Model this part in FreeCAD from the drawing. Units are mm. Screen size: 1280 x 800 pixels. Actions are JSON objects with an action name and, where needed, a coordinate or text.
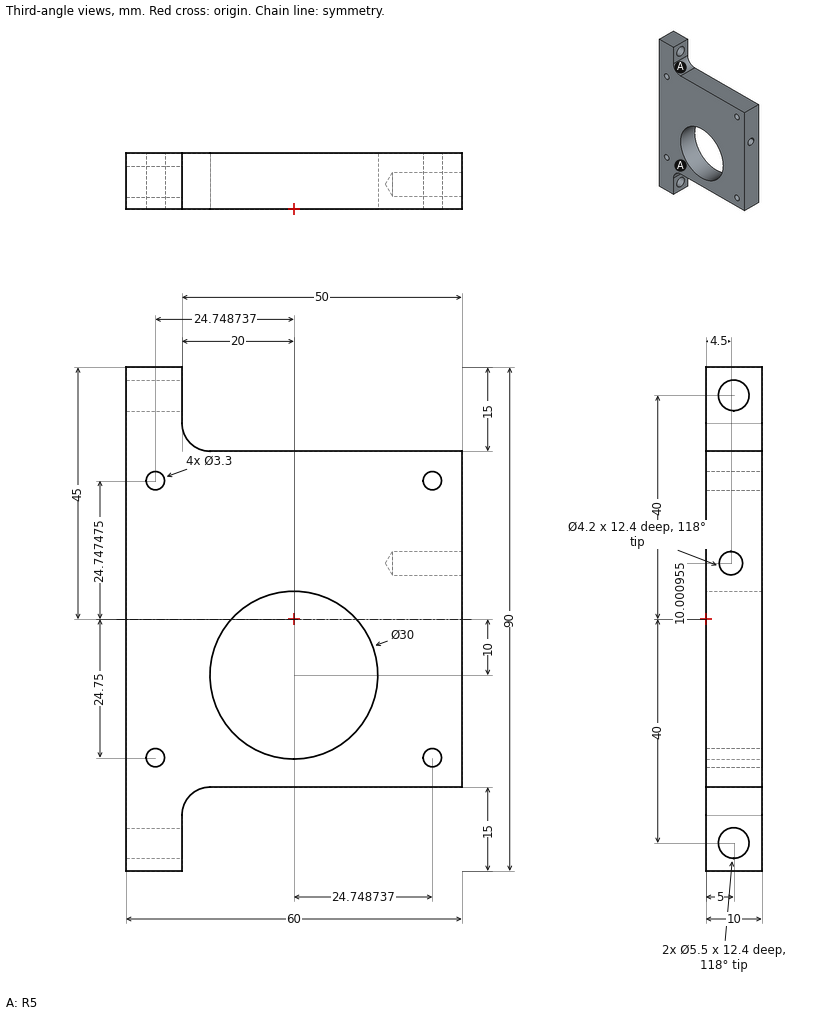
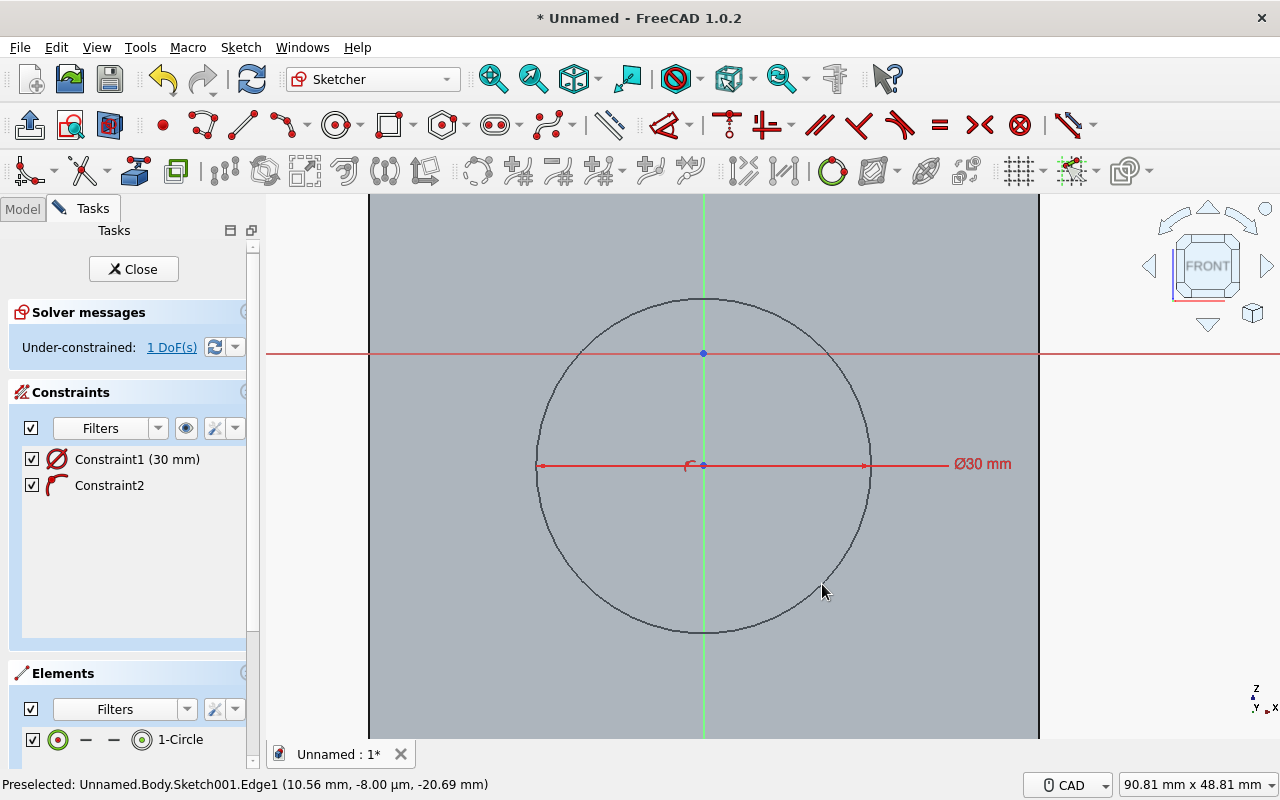
{"action": "left_click", "coordinate": [664, 126]}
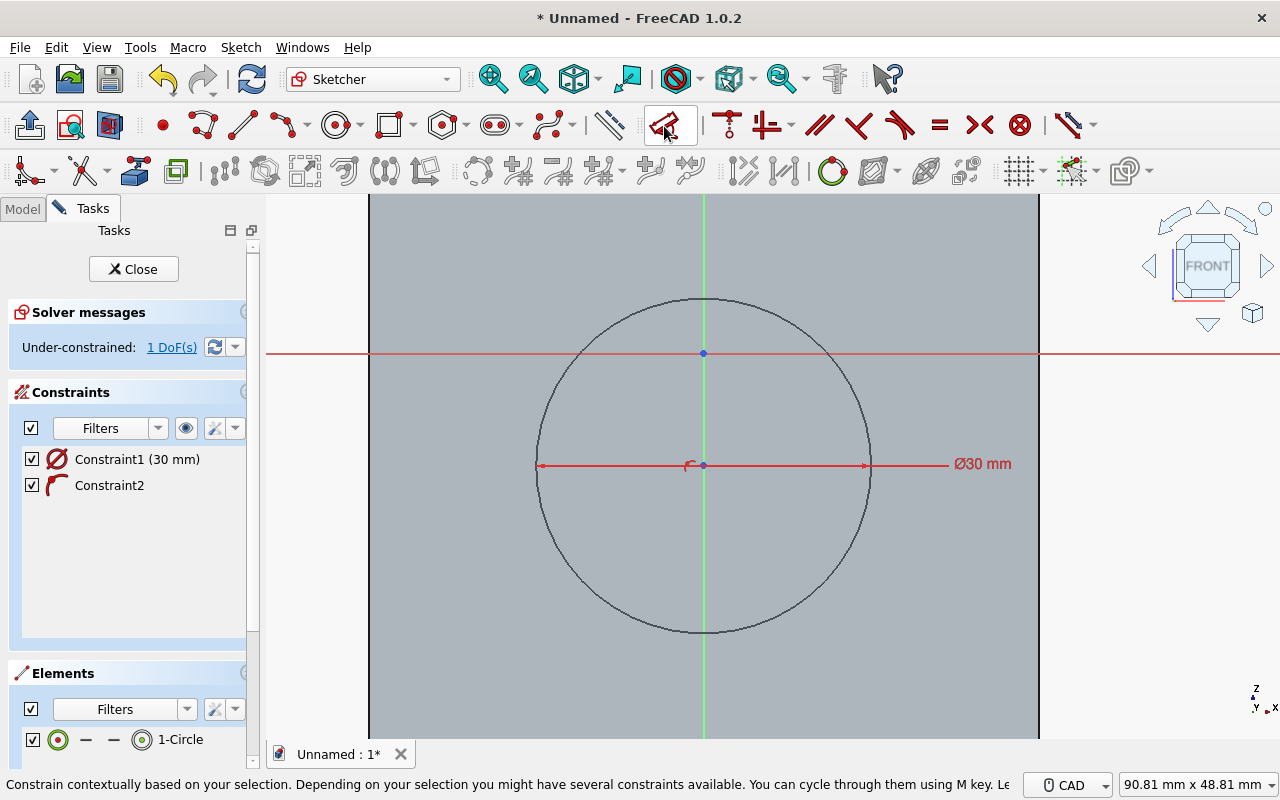
{"action": "left_click", "coordinate": [704, 466]}
{"action": "left_click", "coordinate": [738, 410]}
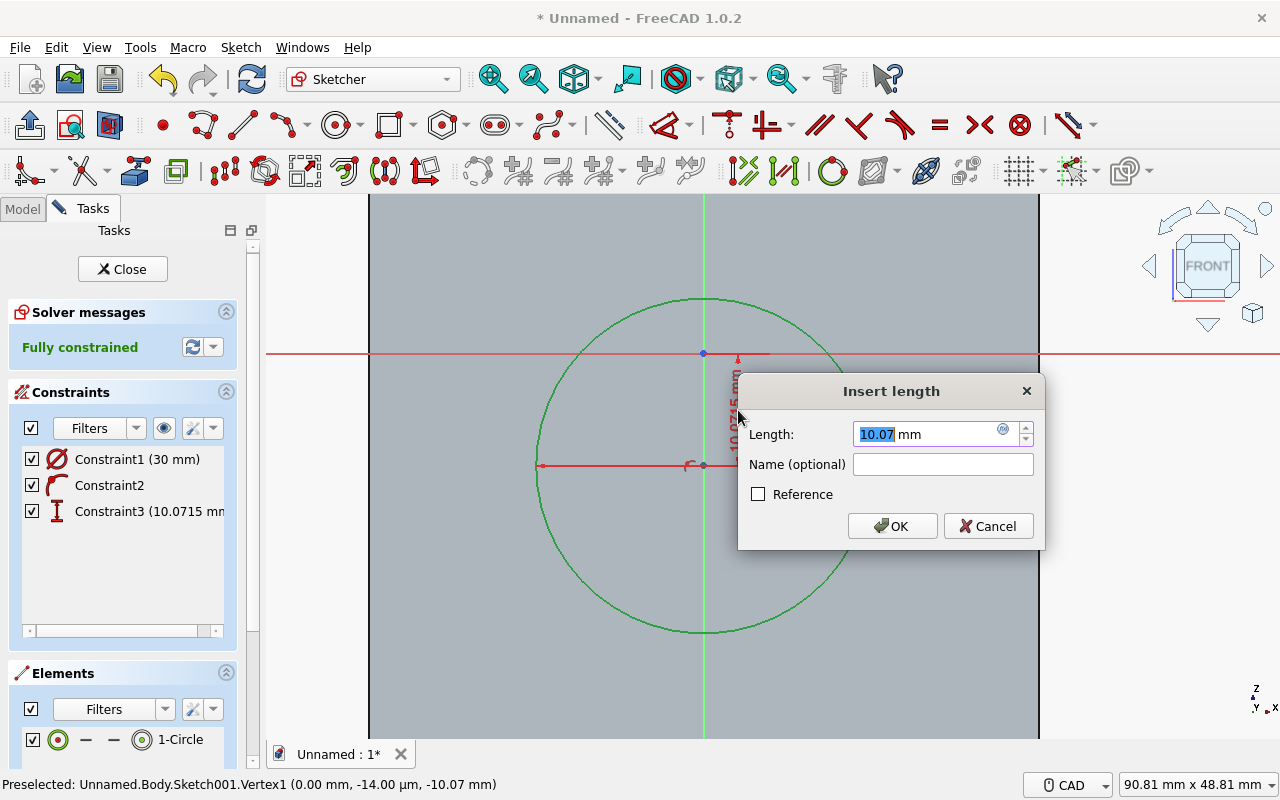
{"action": "type", "text": "10"}
{"action": "key", "text": "Return"}
{"action": "key", "text": "Escape"}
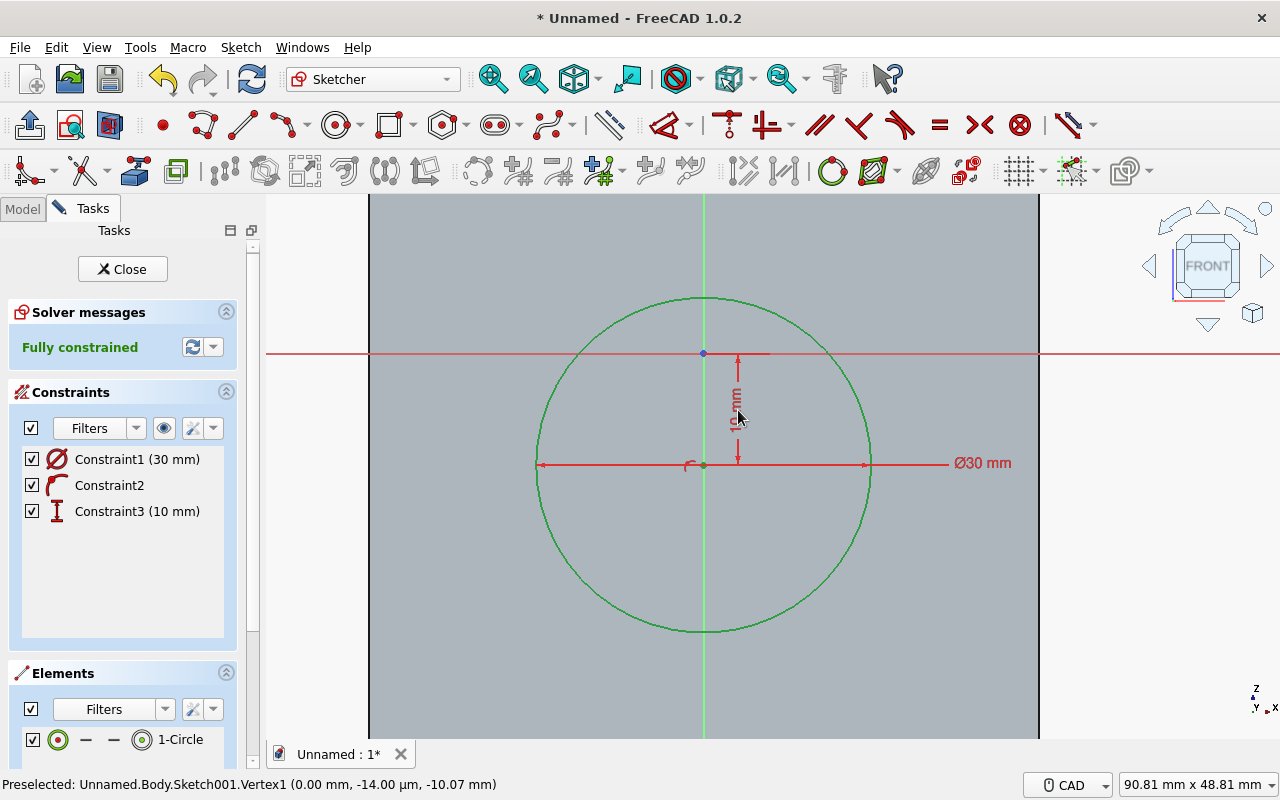
{"action": "left_click", "coordinate": [123, 269]}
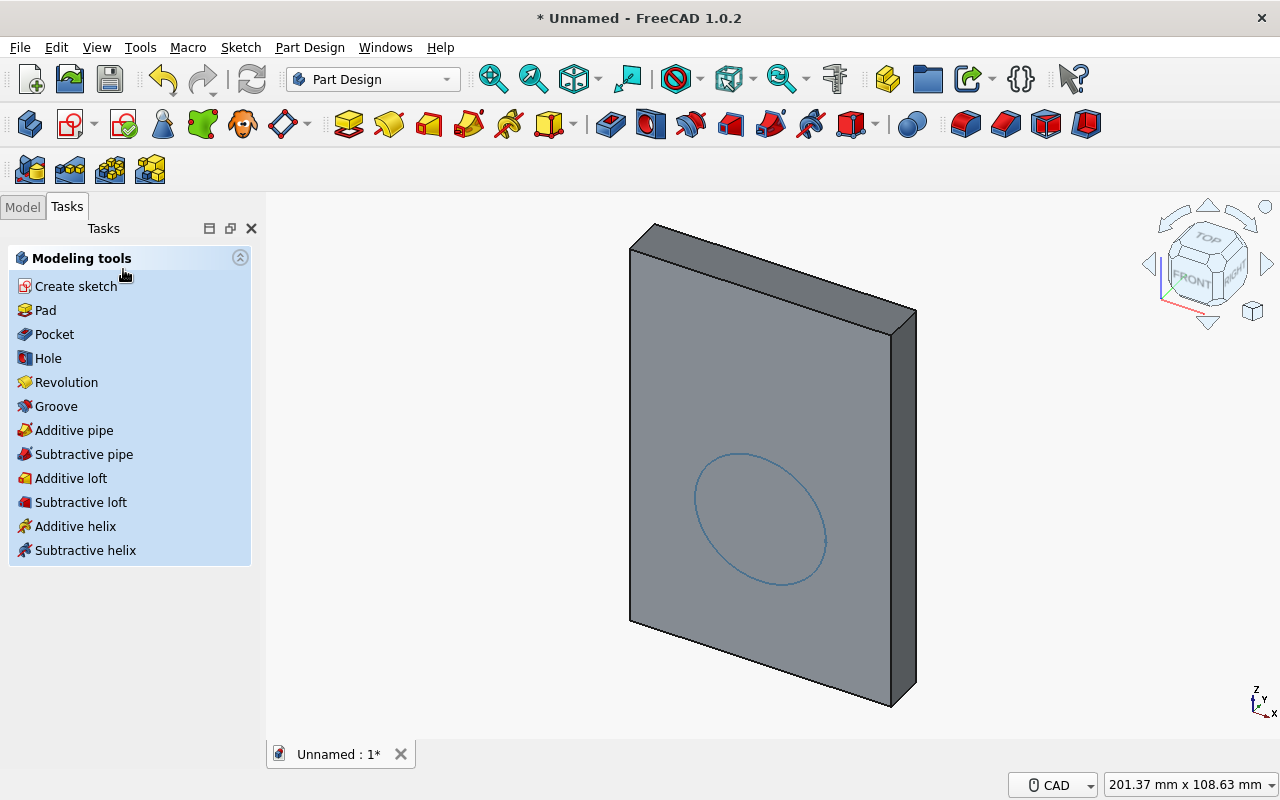
{"action": "left_click", "coordinate": [612, 124]}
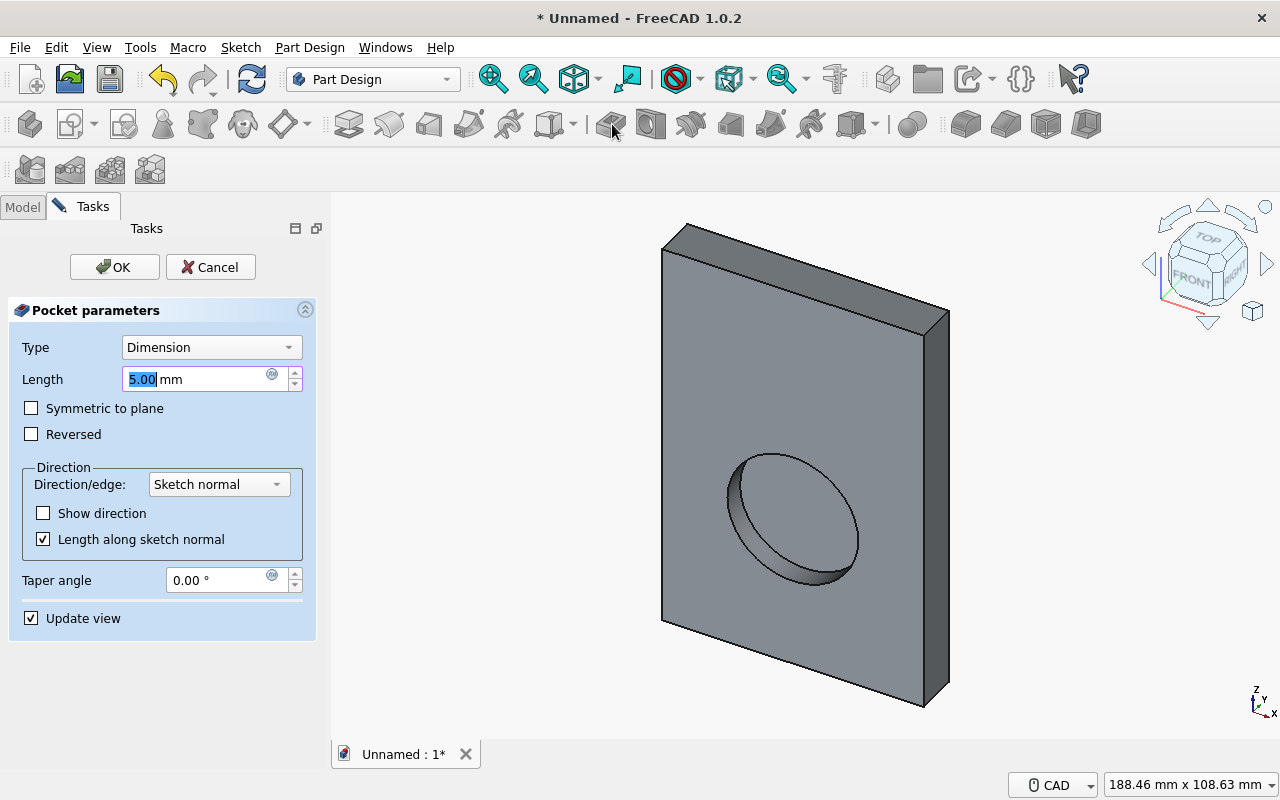
{"action": "left_click", "coordinate": [212, 348]}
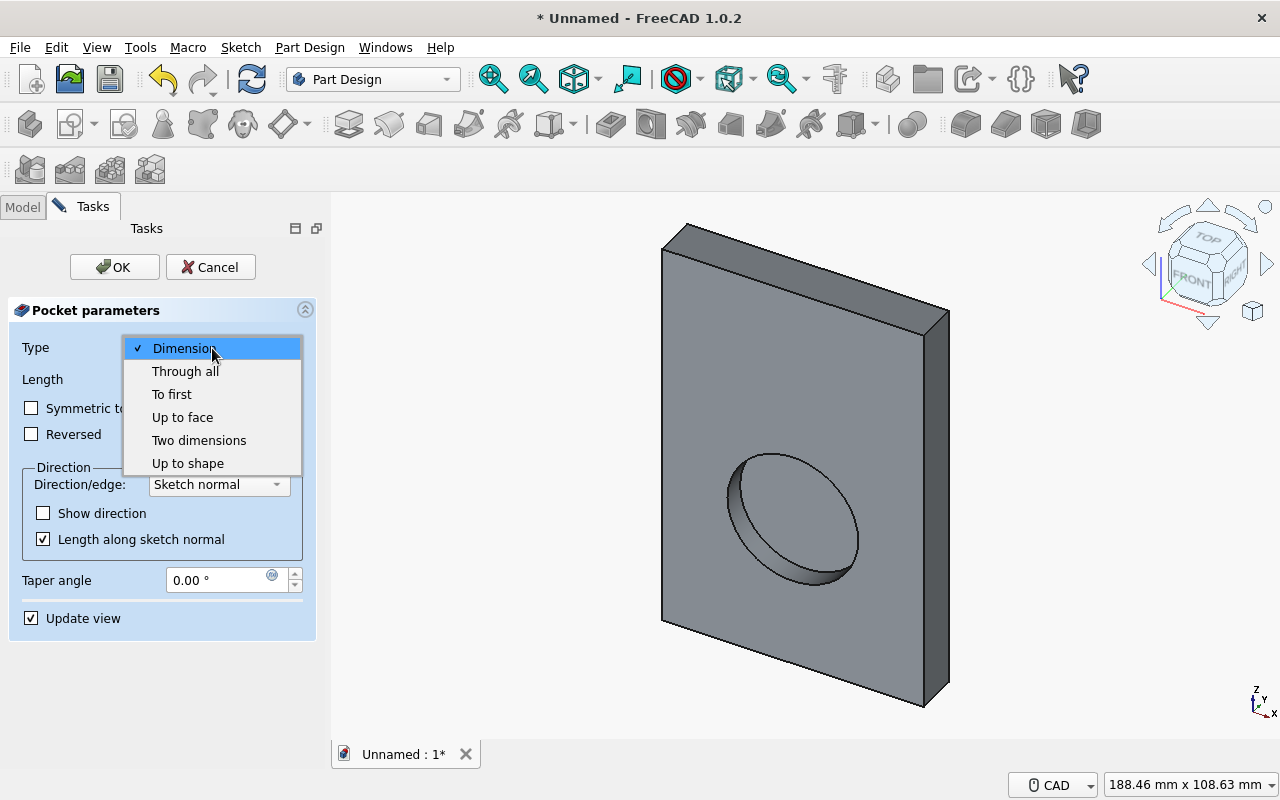
{"action": "left_click", "coordinate": [212, 372]}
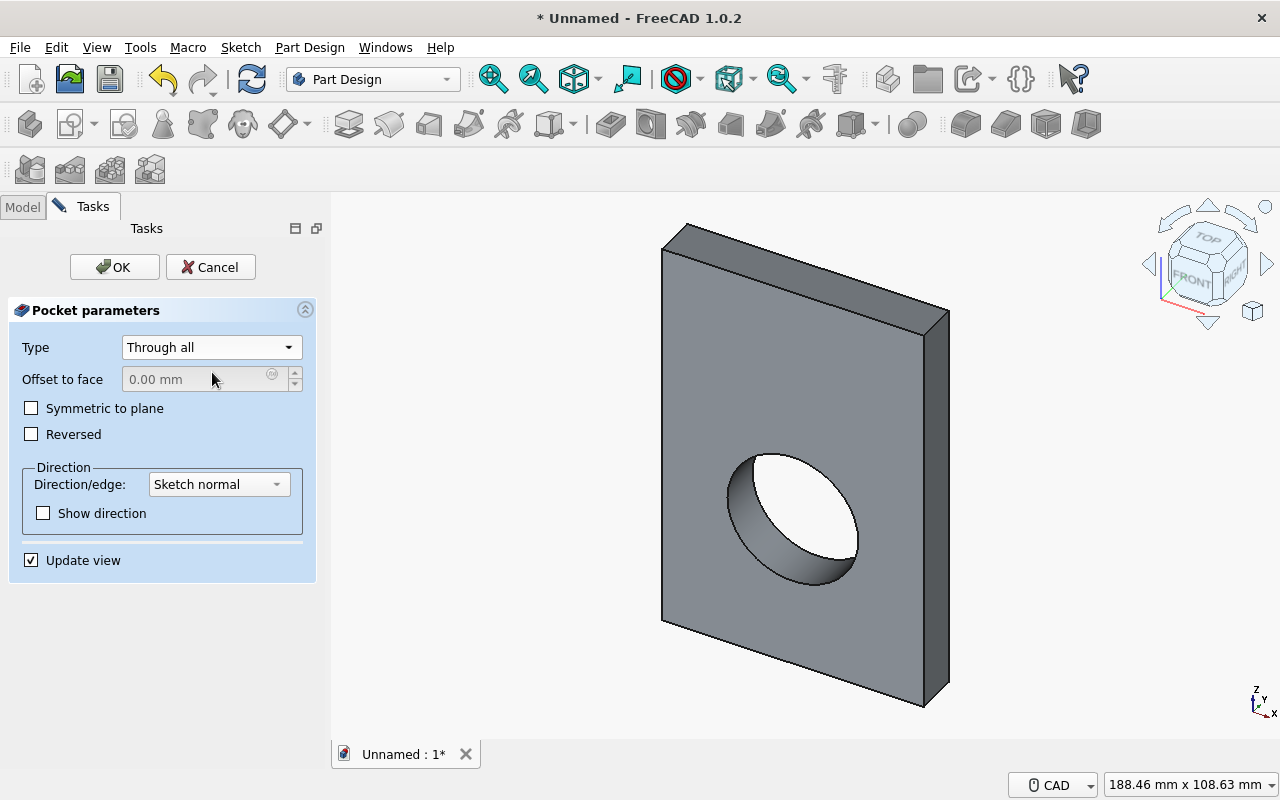
{"action": "left_click", "coordinate": [115, 267]}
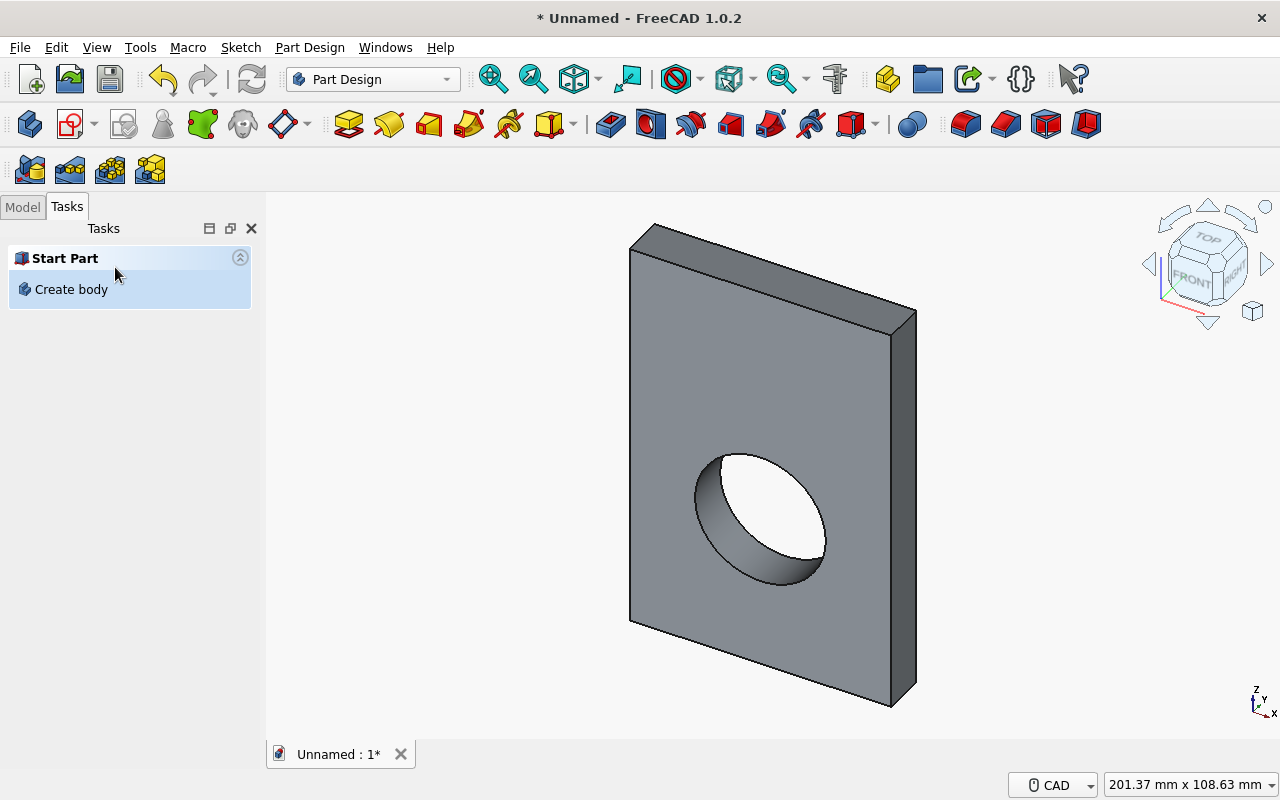
{"action": "left_click", "coordinate": [798, 383]}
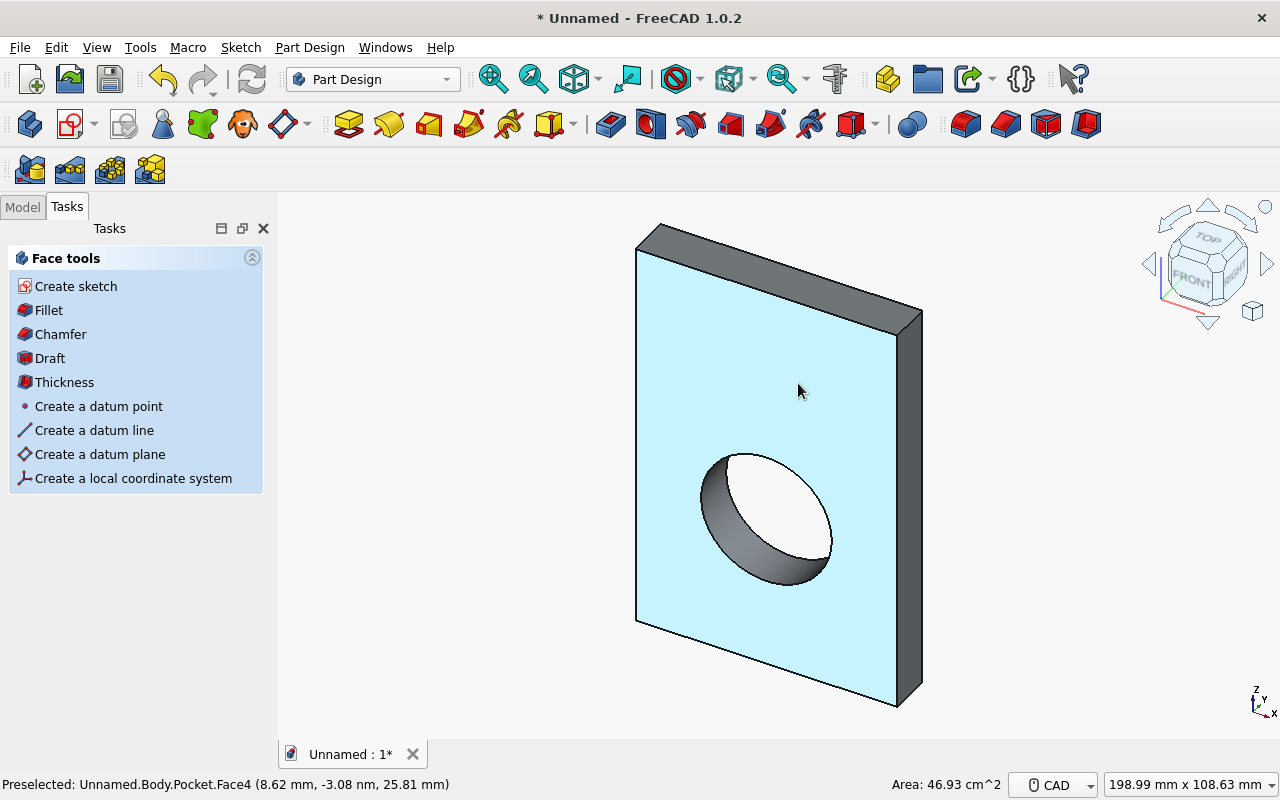
{"action": "left_click", "coordinate": [70, 124]}